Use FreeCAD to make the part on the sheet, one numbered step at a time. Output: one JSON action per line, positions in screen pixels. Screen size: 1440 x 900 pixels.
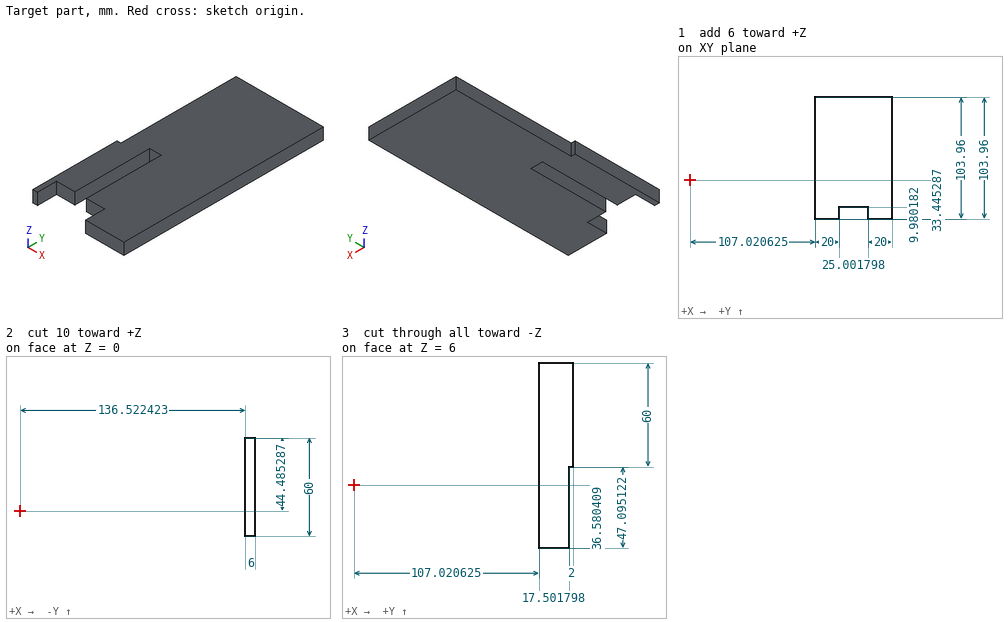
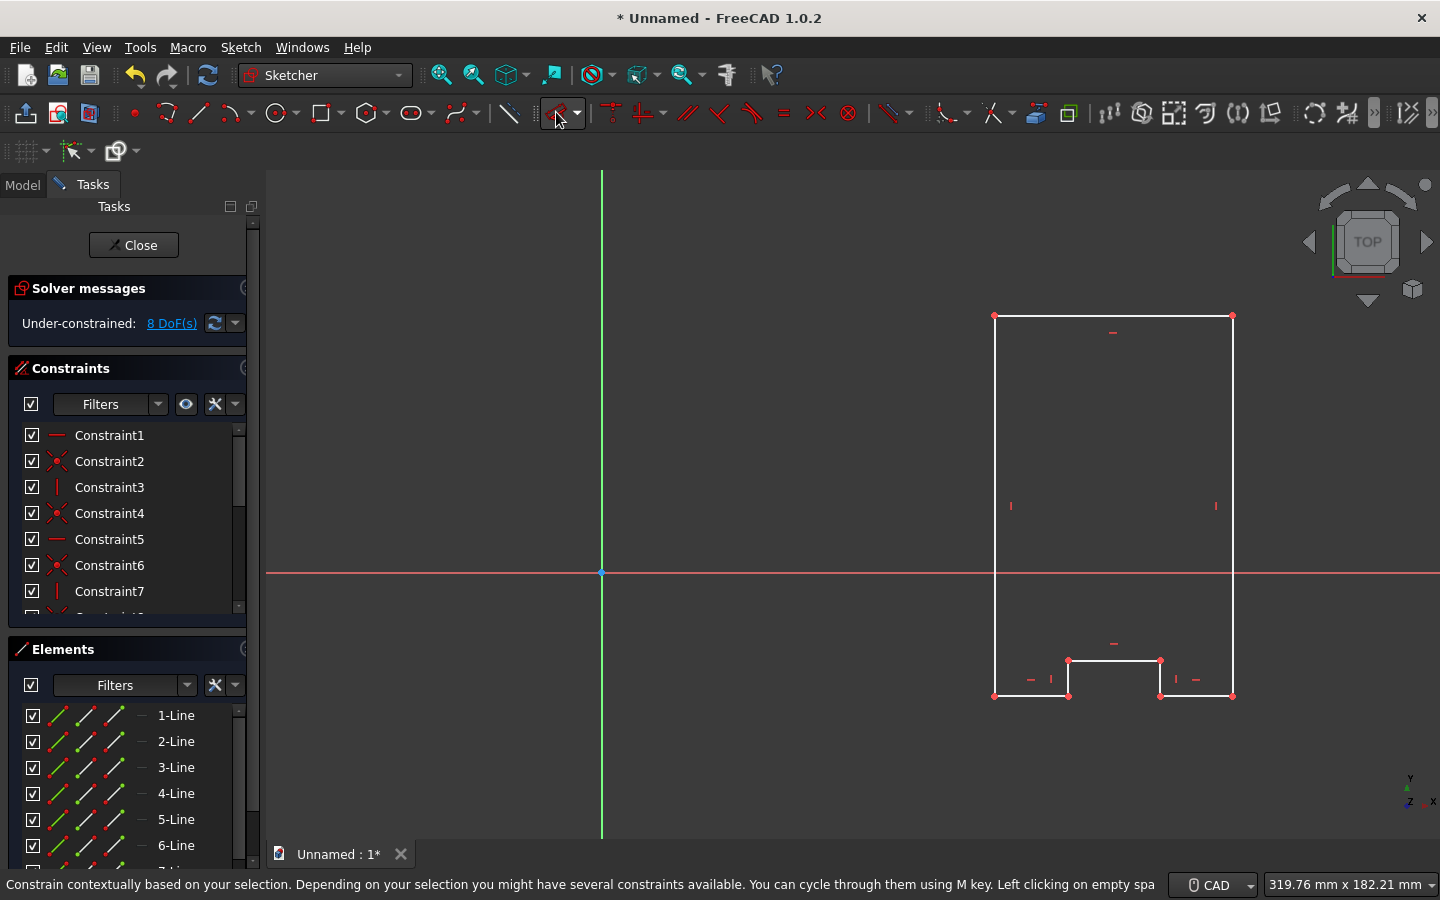
{"action": "left_click", "coordinate": [1017, 696]}
{"action": "left_click", "coordinate": [1031, 730]}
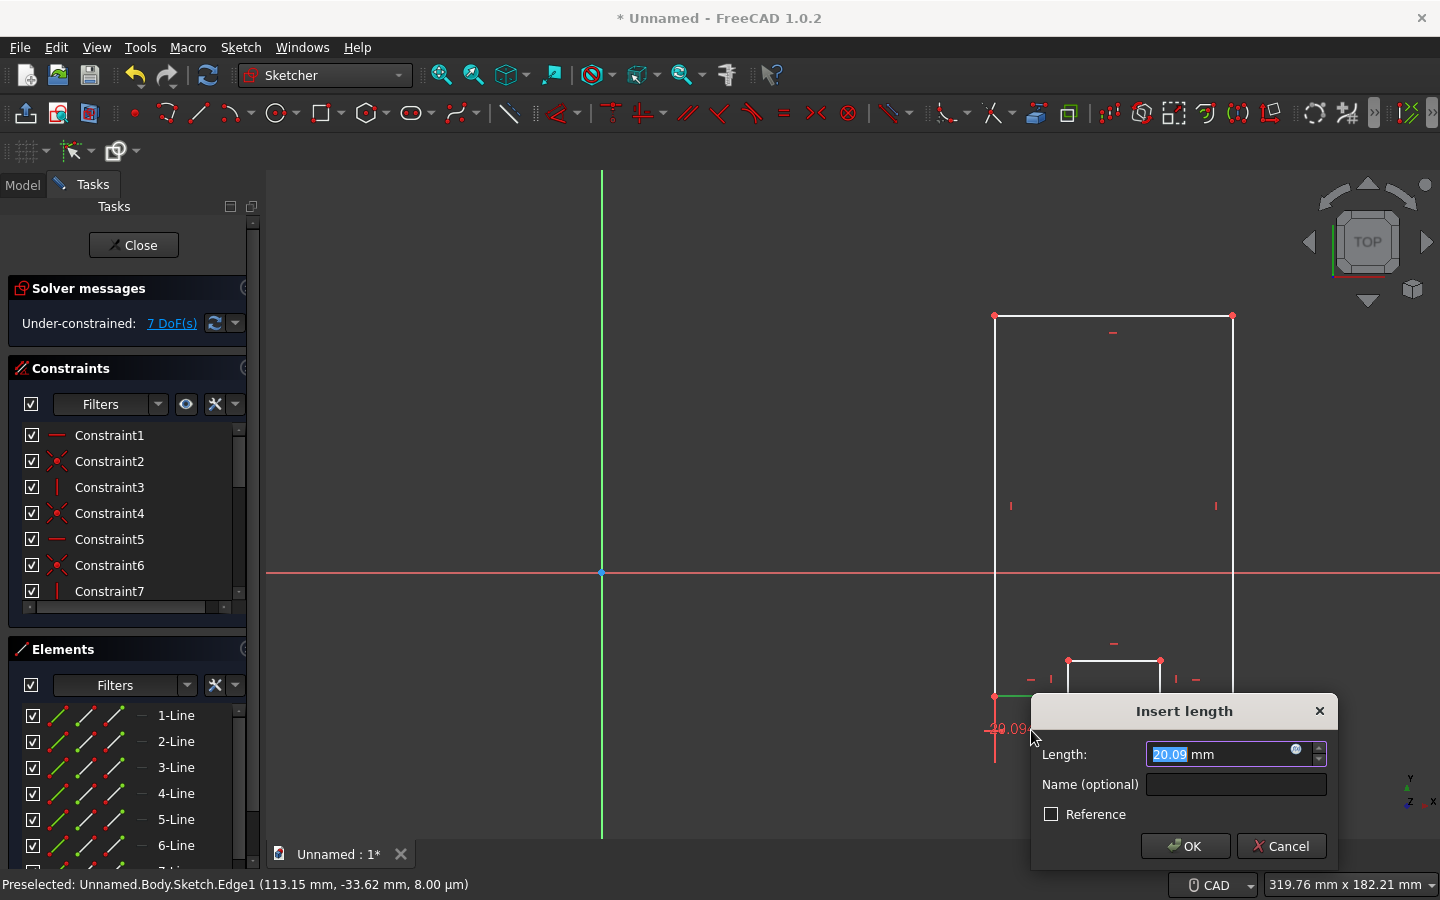
{"action": "type", "text": "20"}
{"action": "key", "text": "Return"}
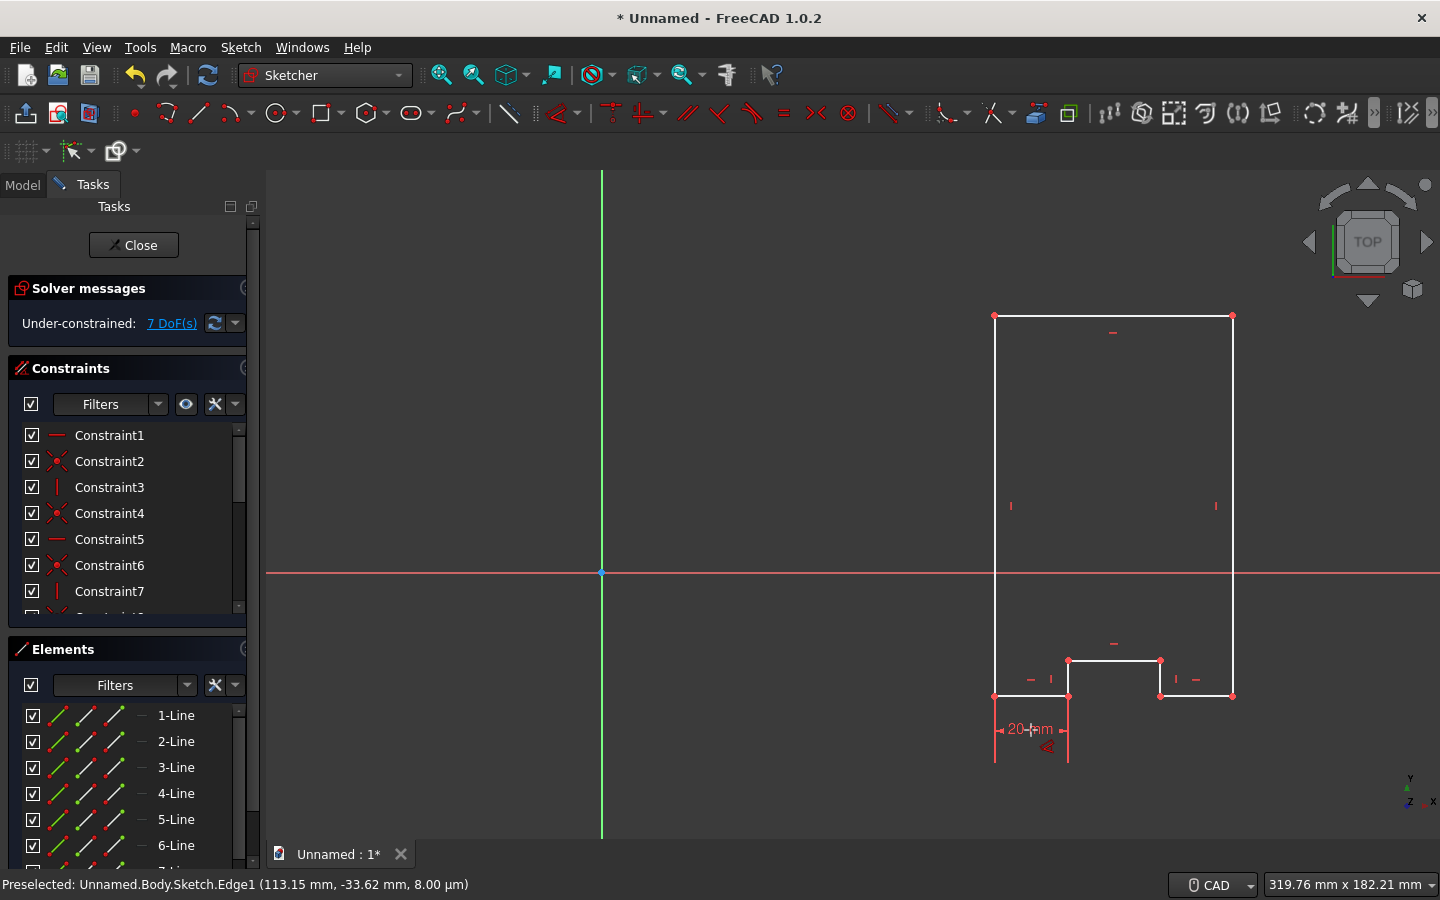
{"action": "left_click", "coordinate": [1182, 696]}
{"action": "left_click", "coordinate": [1196, 730]}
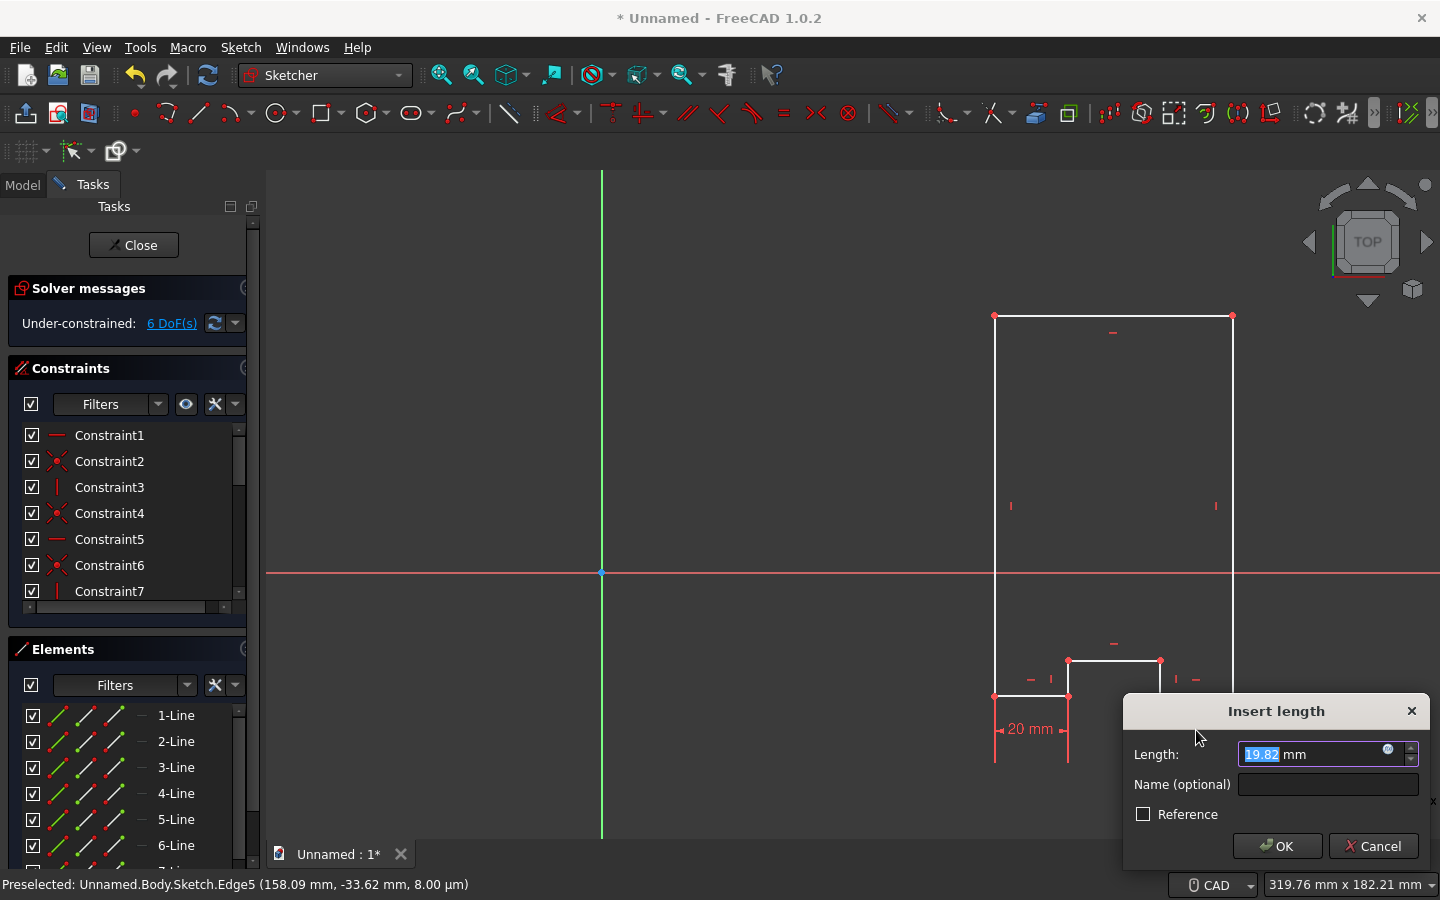
{"action": "type", "text": "20"}
{"action": "key", "text": "Return"}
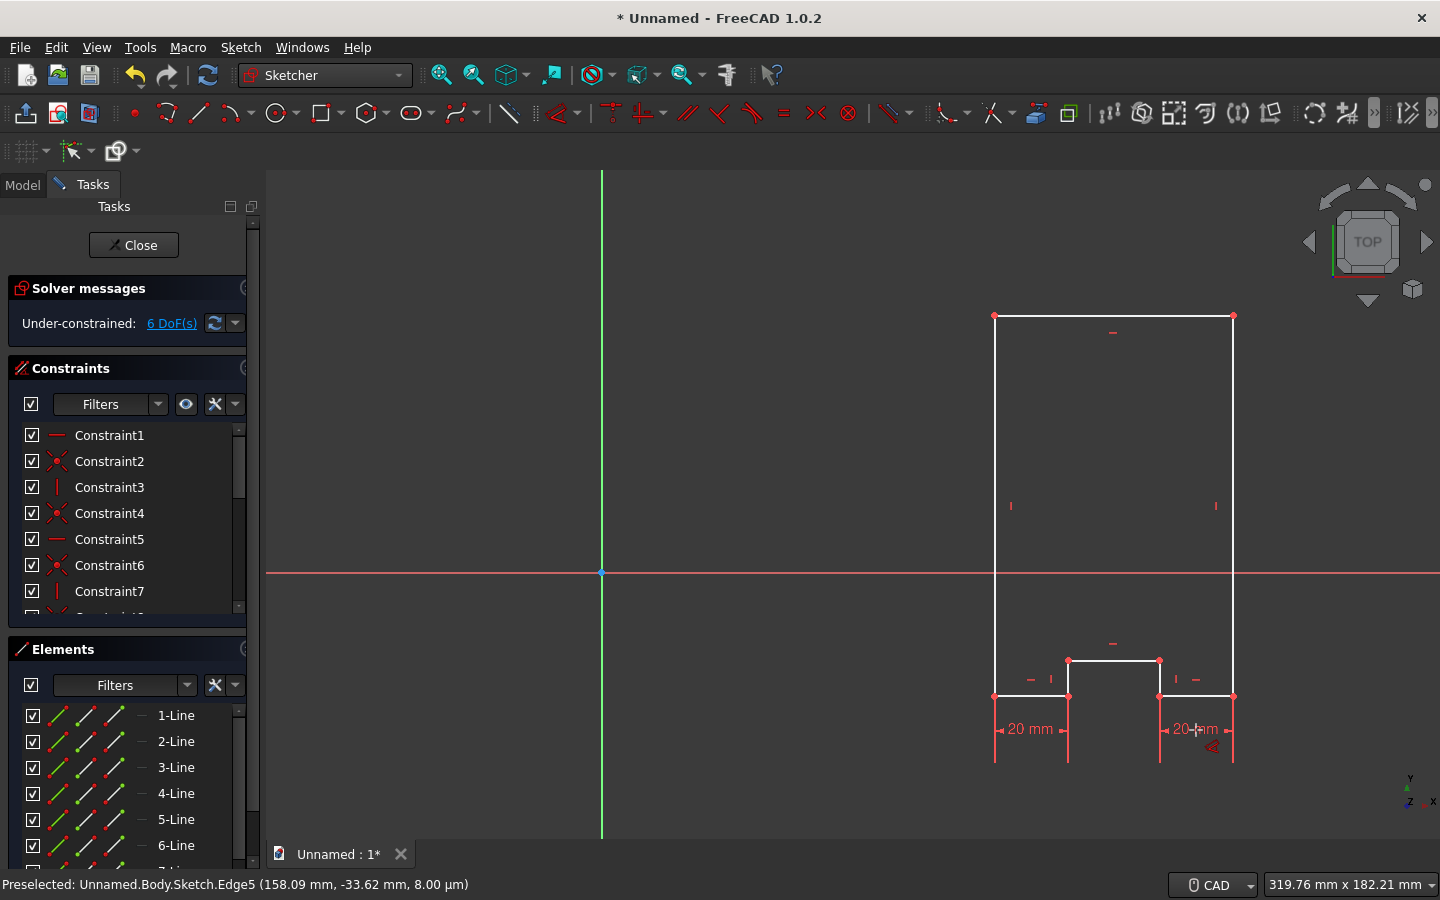
{"action": "scroll", "coordinate": [1233, 582], "scroll_direction": "up", "scroll_amount": 3}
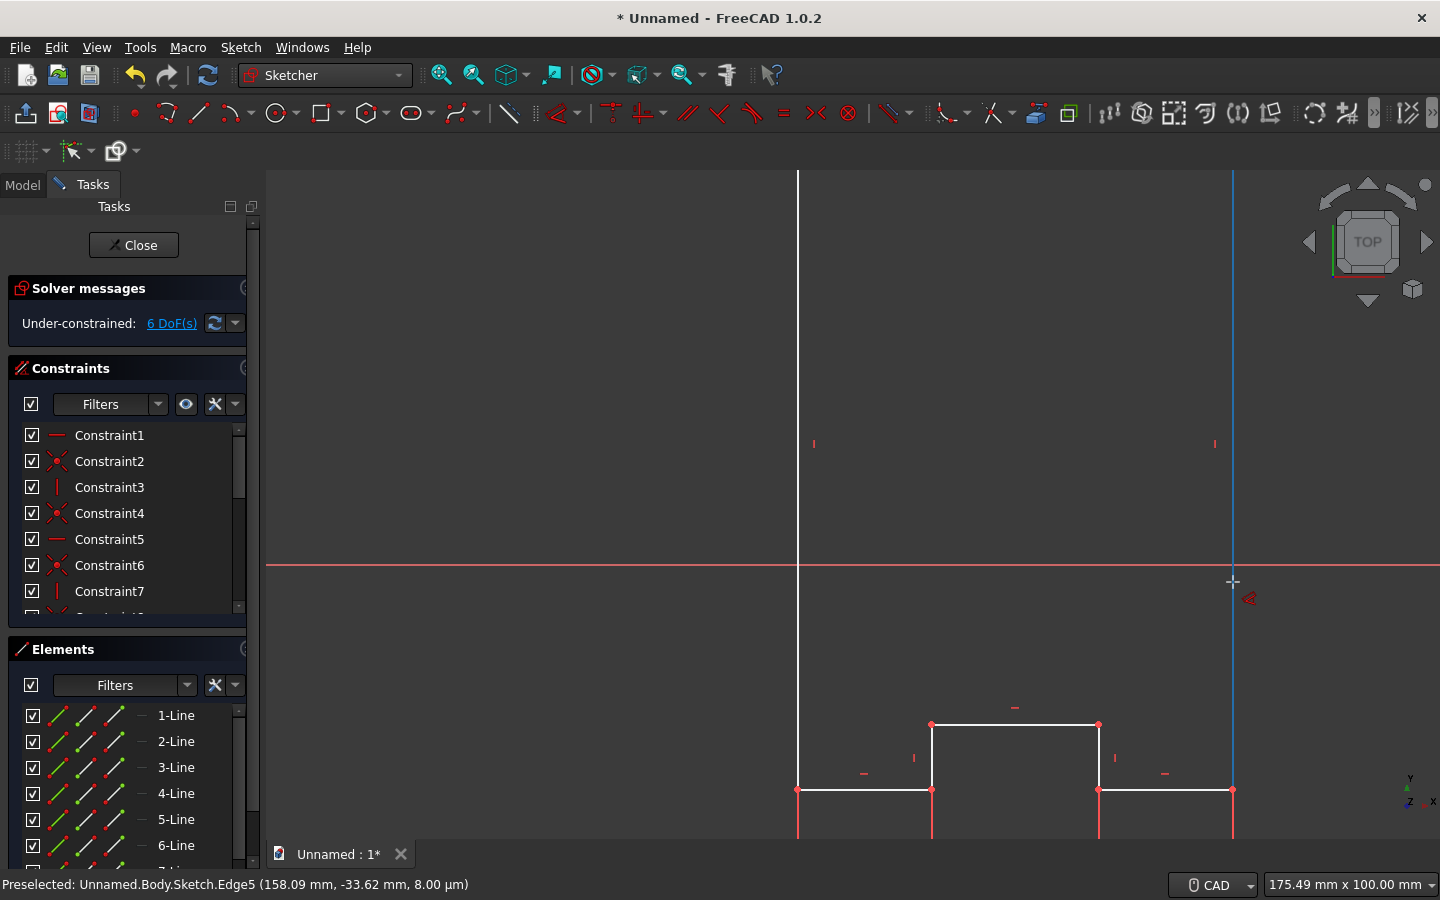
{"action": "left_click", "coordinate": [1233, 582]}
{"action": "left_click", "coordinate": [1267, 494]}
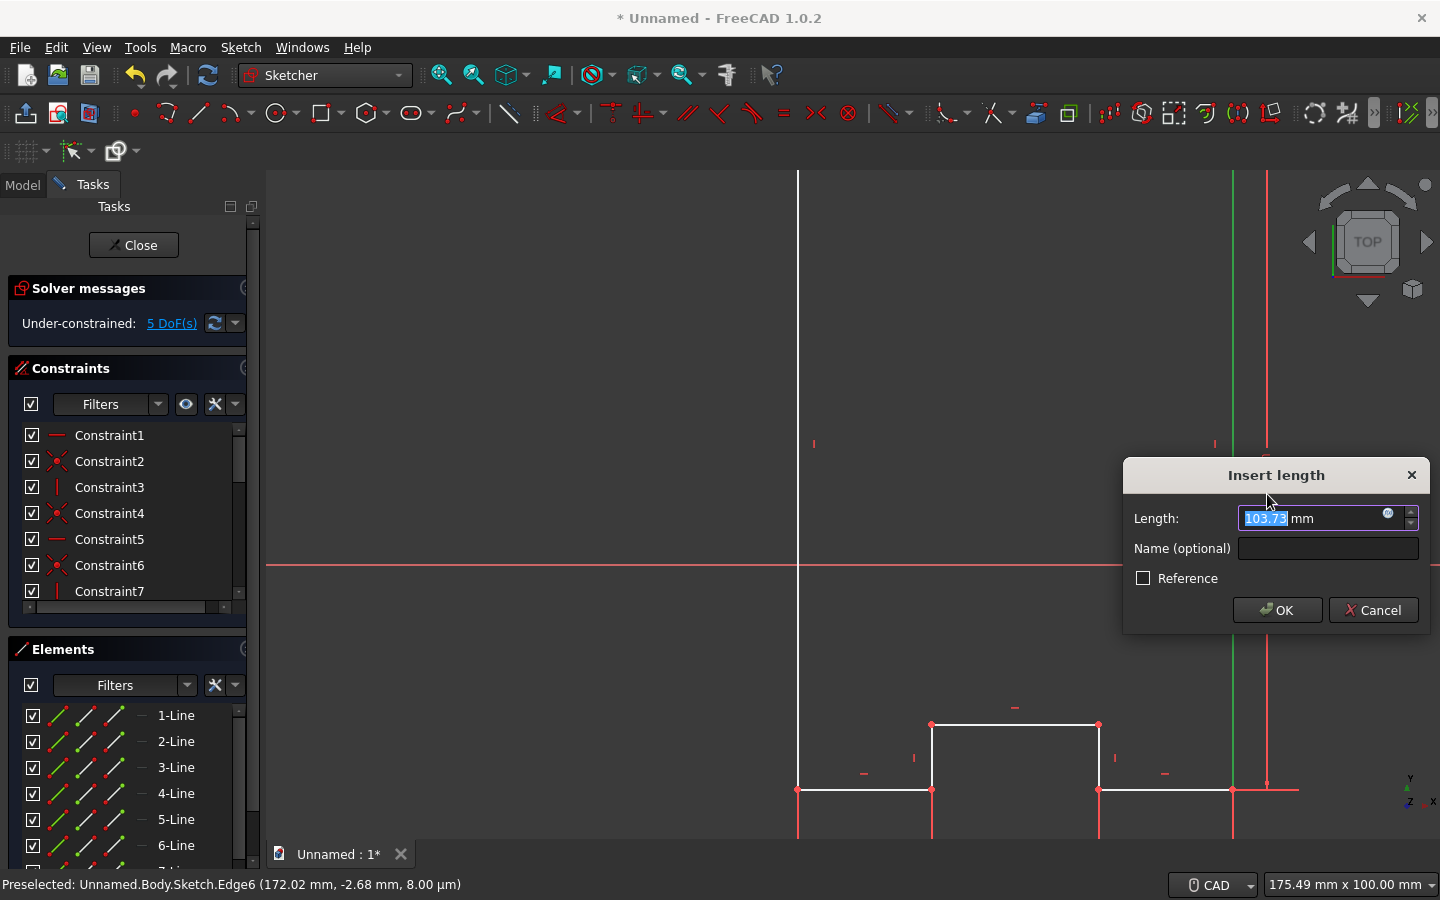
{"action": "type", "text": "103.96"}
{"action": "key", "text": "Return"}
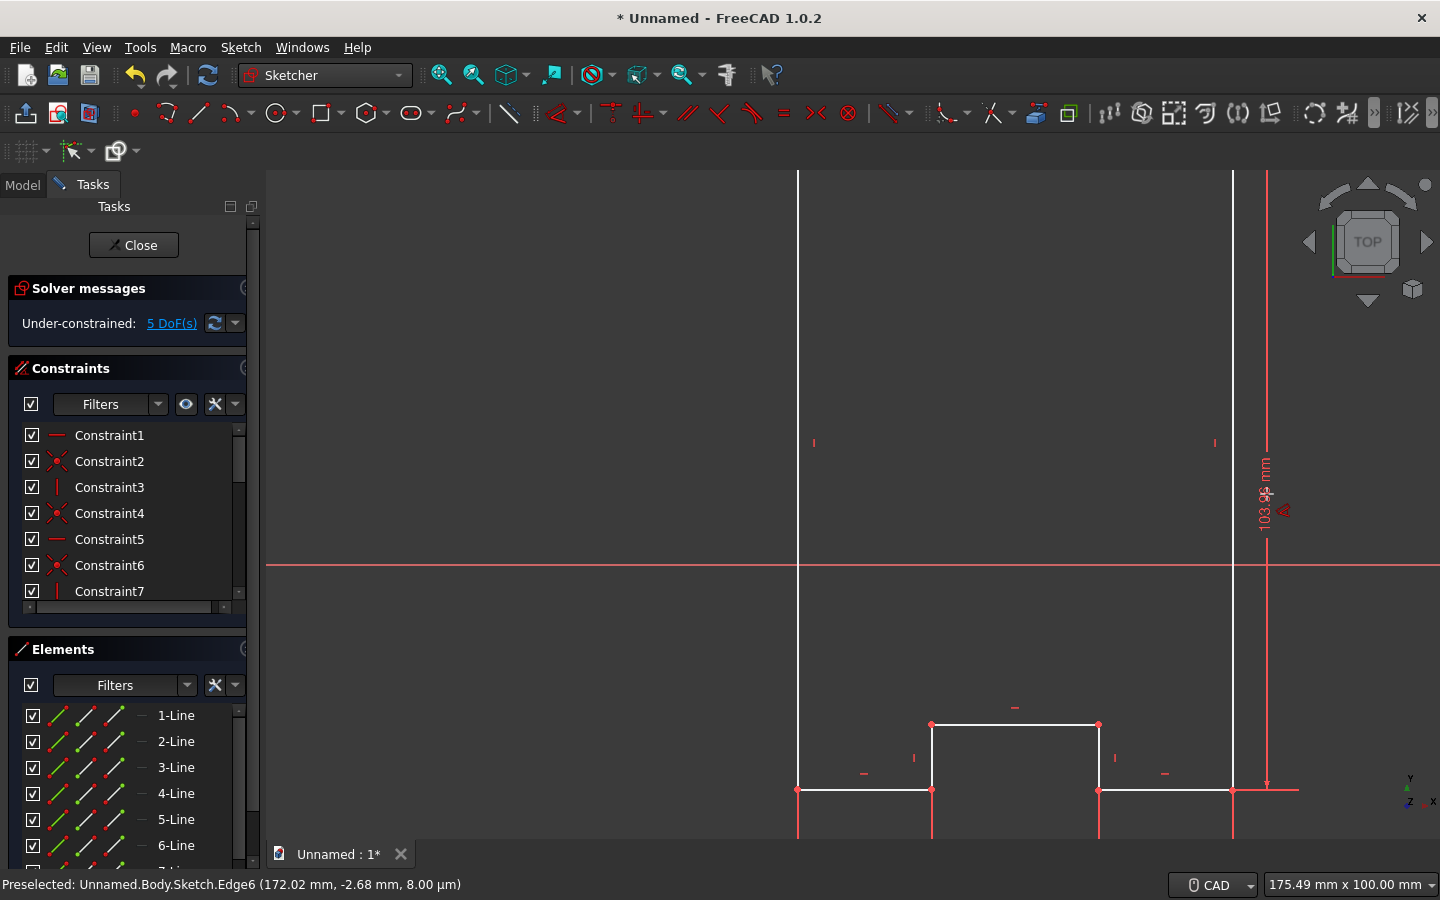
{"action": "left_click", "coordinate": [798, 303]}
{"action": "left_click", "coordinate": [832, 494]}